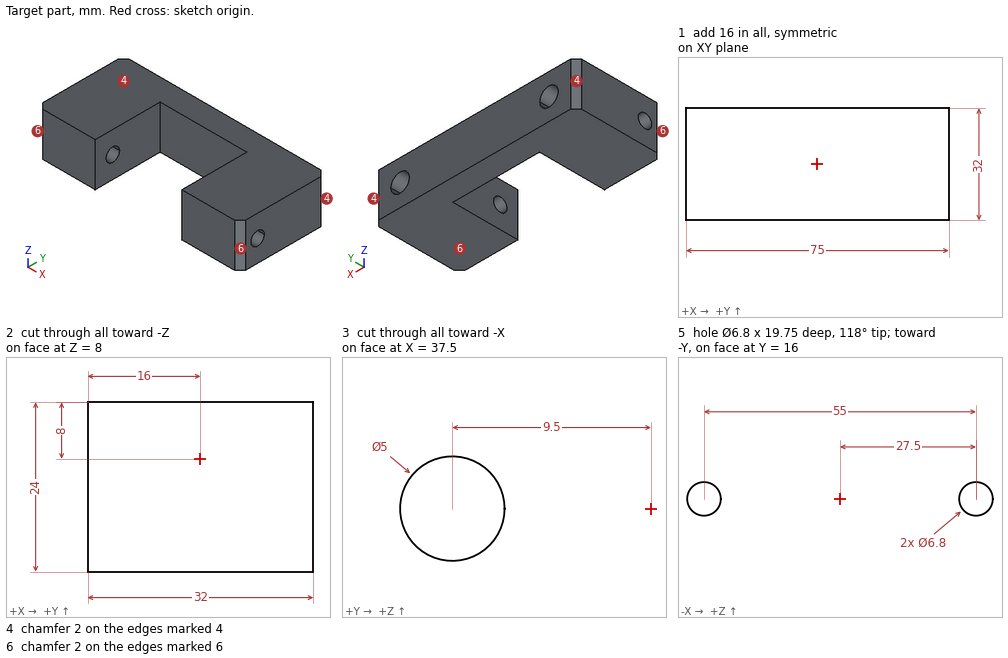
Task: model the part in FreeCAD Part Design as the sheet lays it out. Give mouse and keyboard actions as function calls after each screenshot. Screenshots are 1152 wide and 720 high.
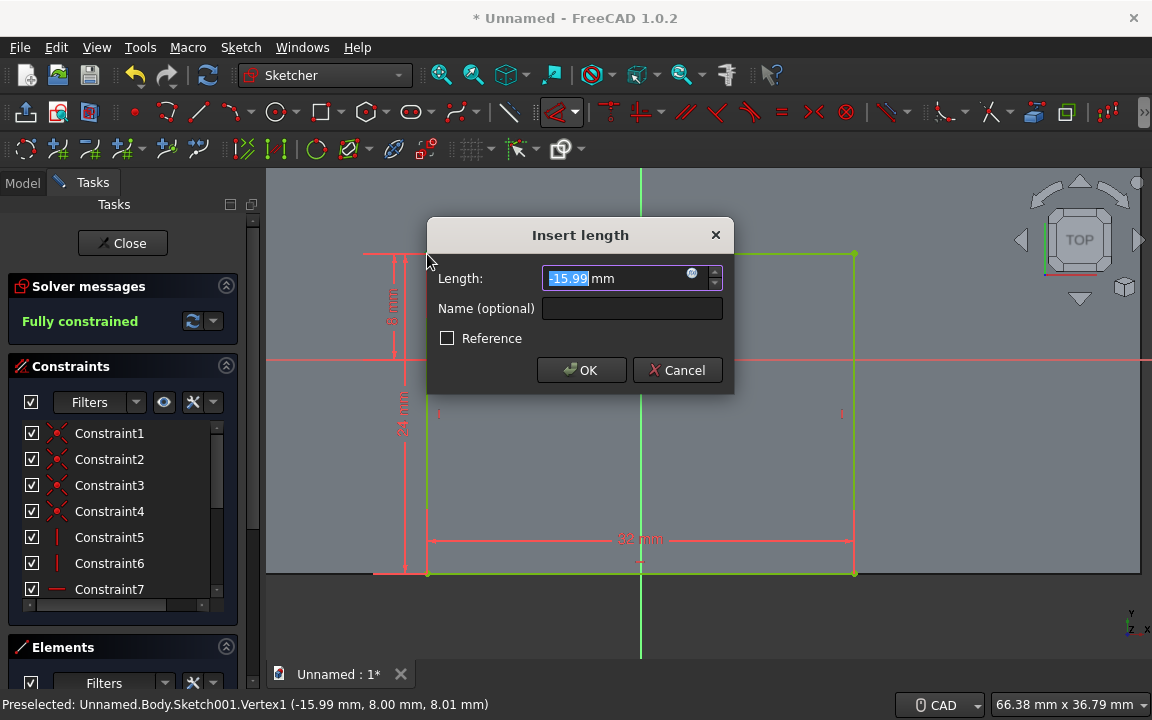
text(-16)
key(Return)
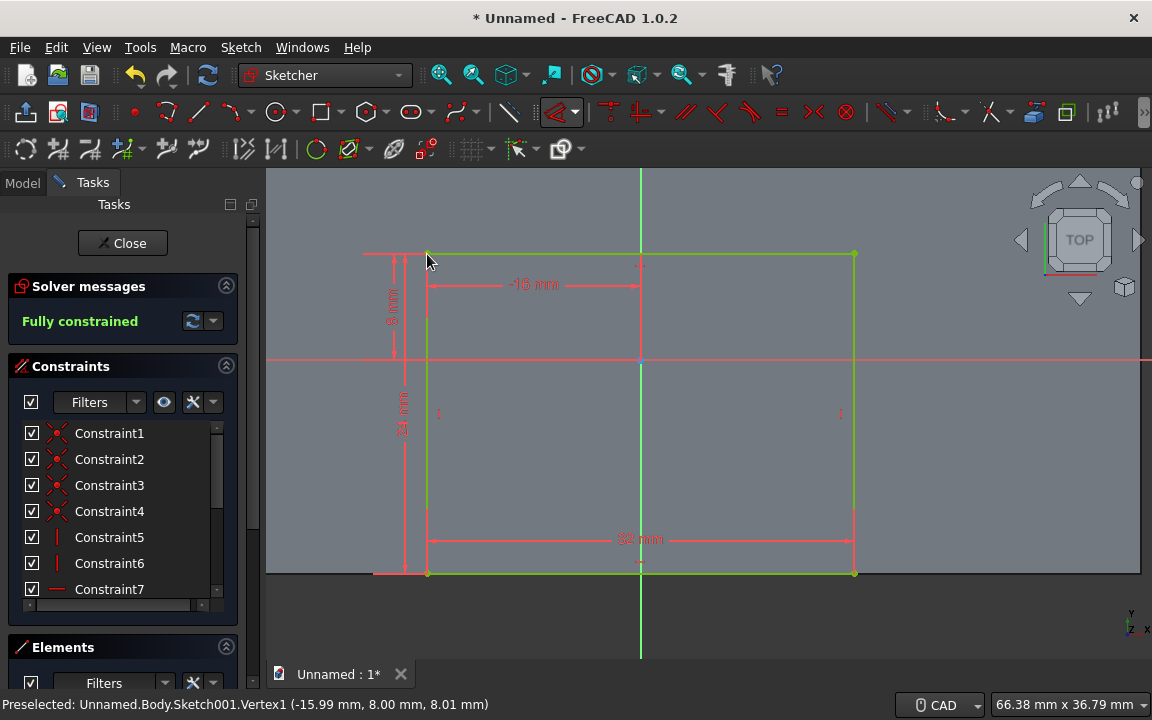
click(123, 243)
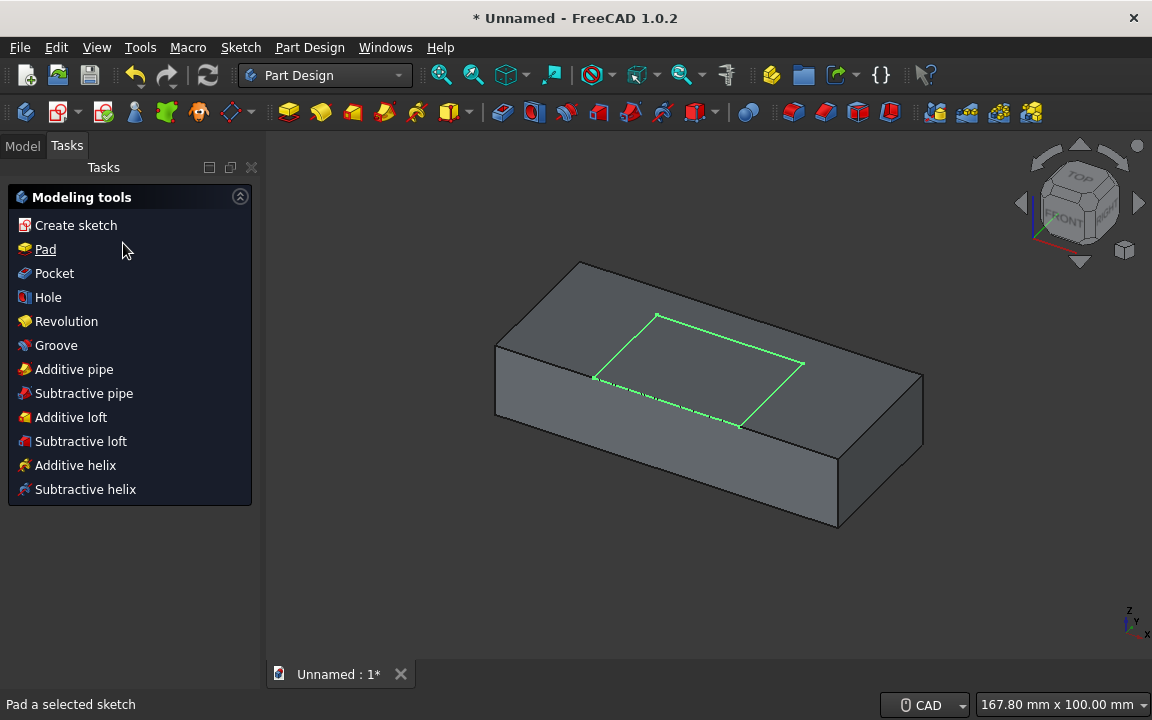
click(504, 112)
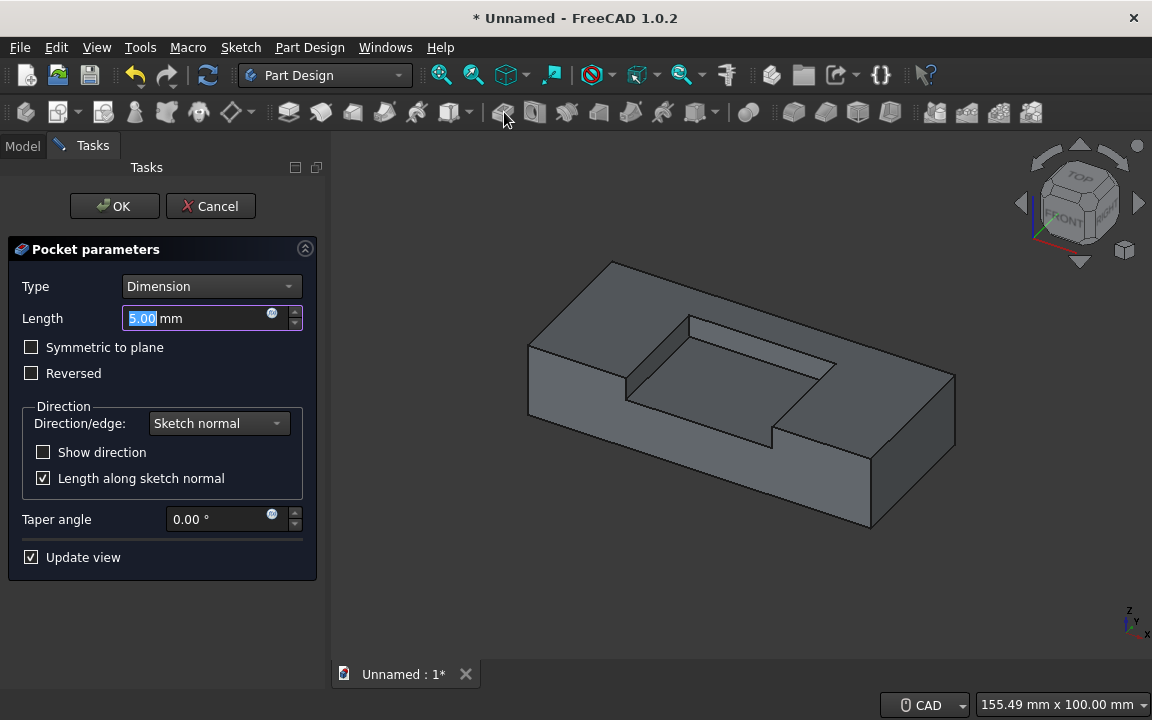
click(212, 286)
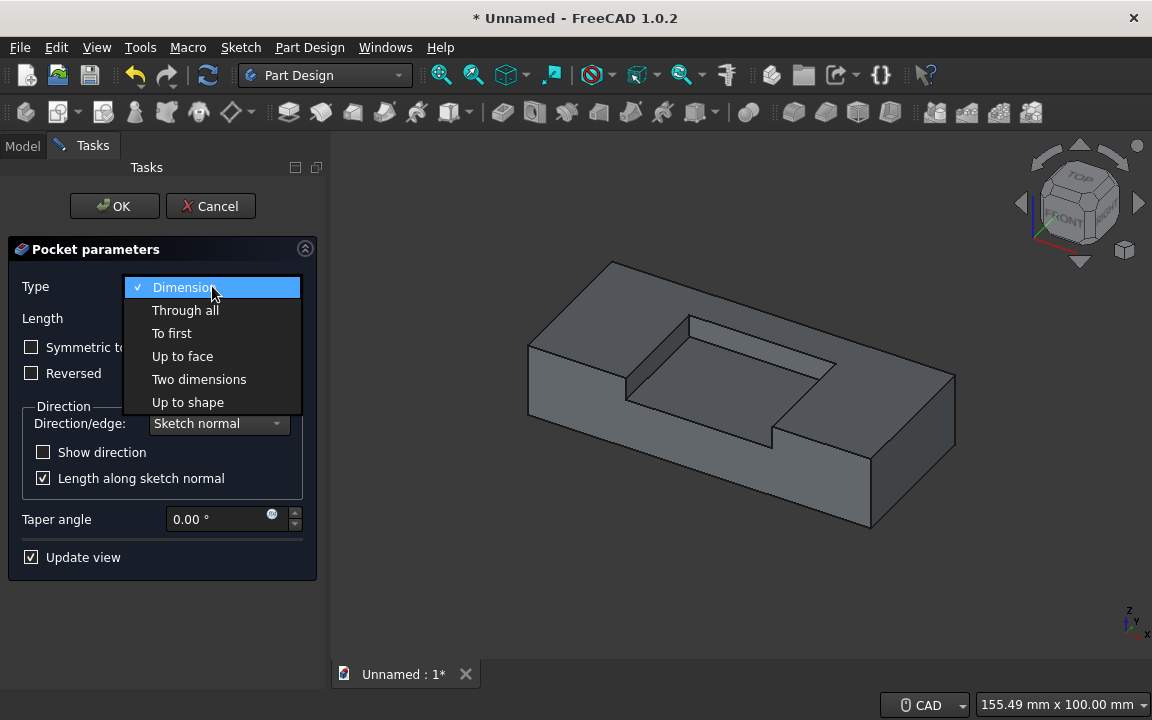
click(212, 310)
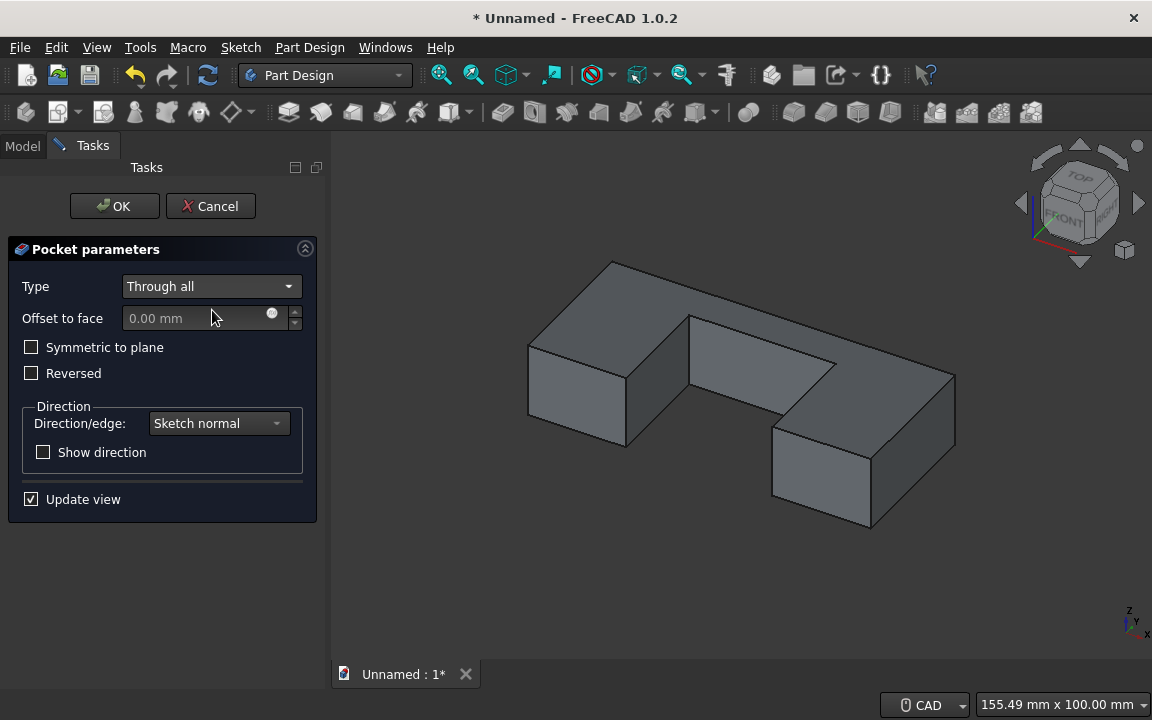
click(115, 206)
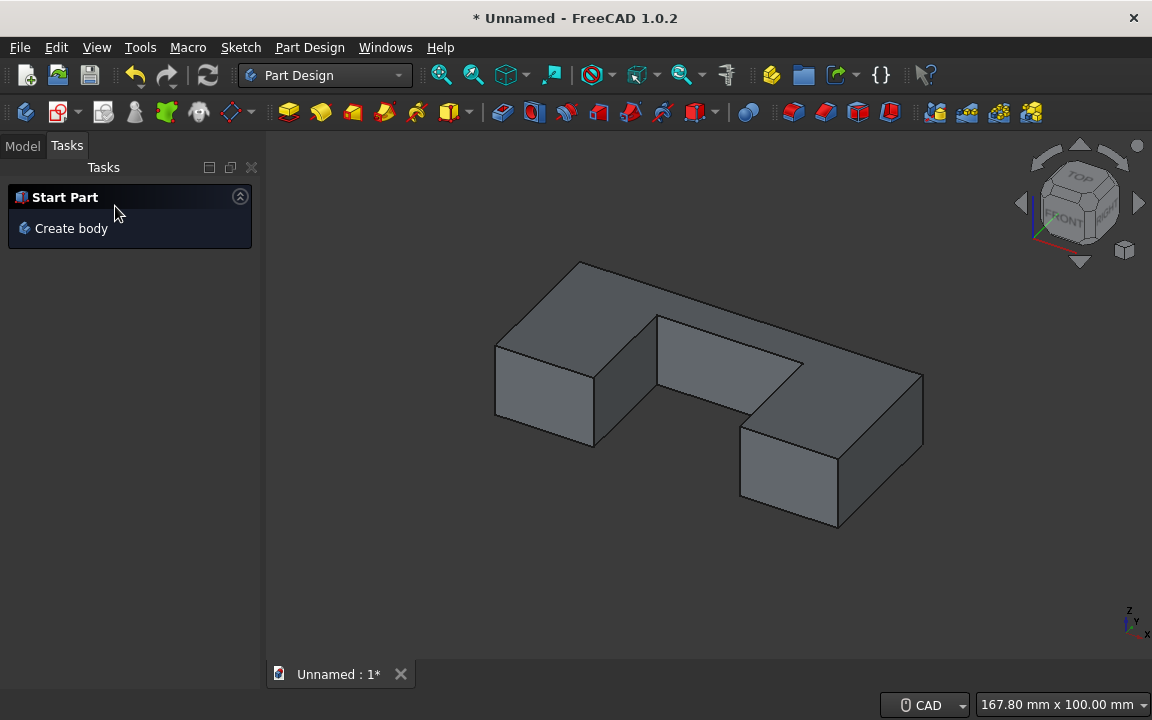
click(893, 439)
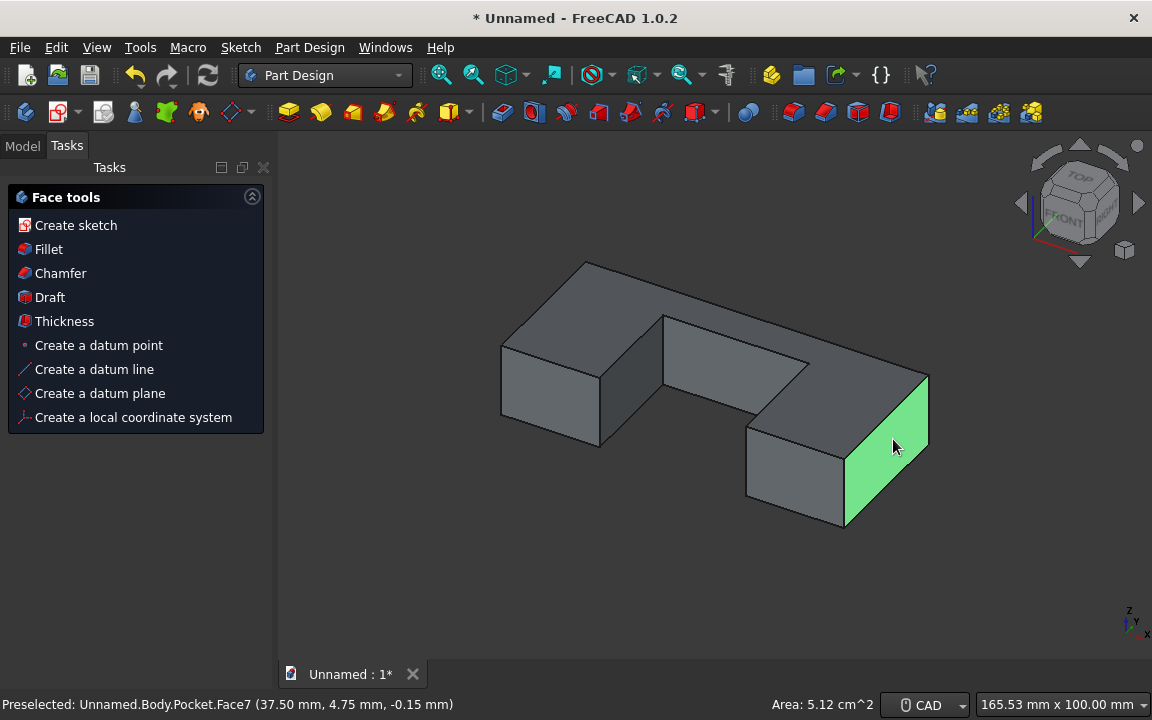
click(58, 112)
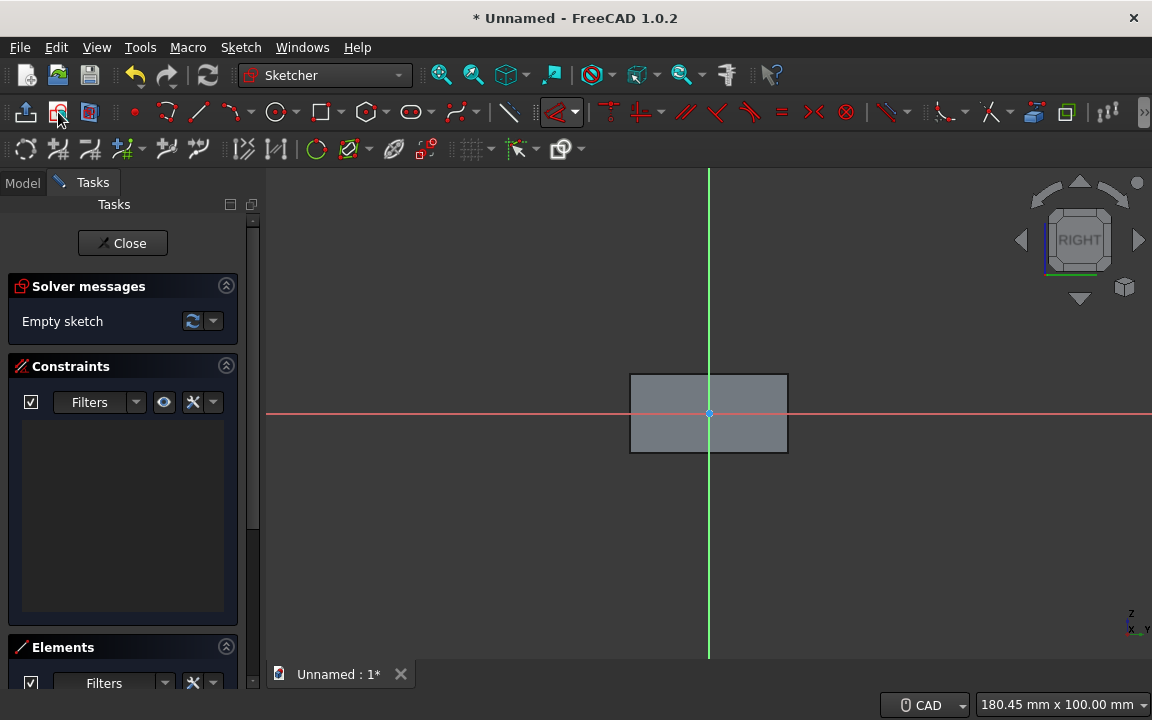
scroll(684, 414, up, 11)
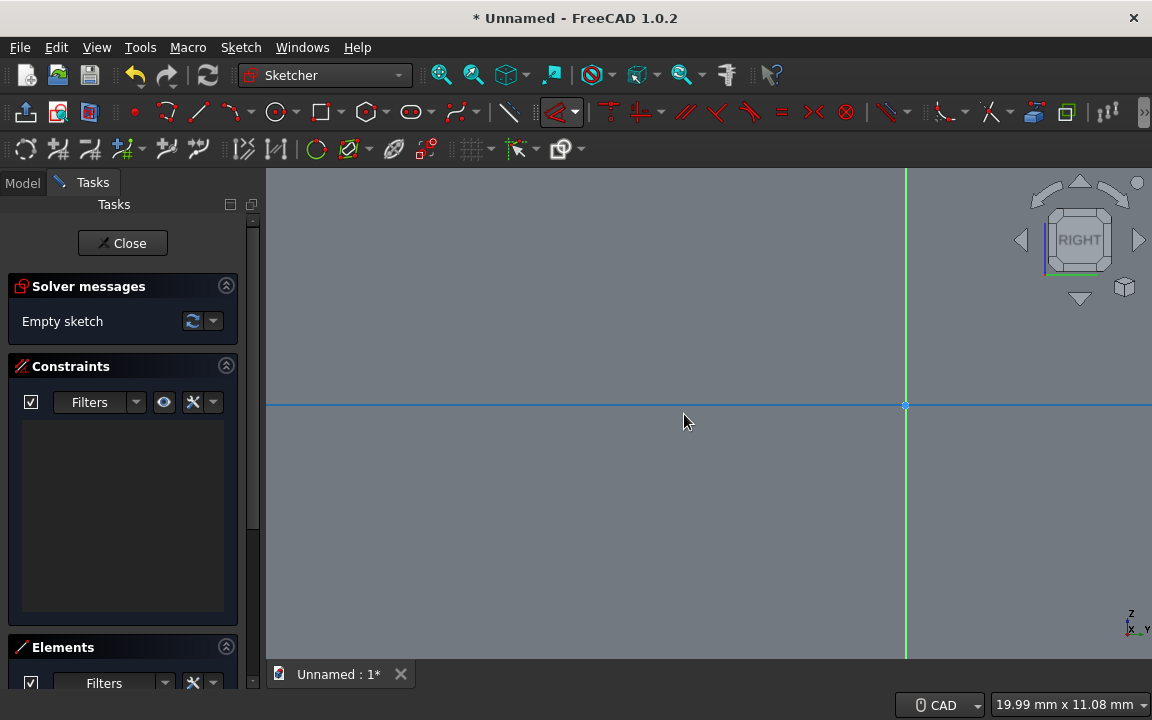
key(g)
key(c)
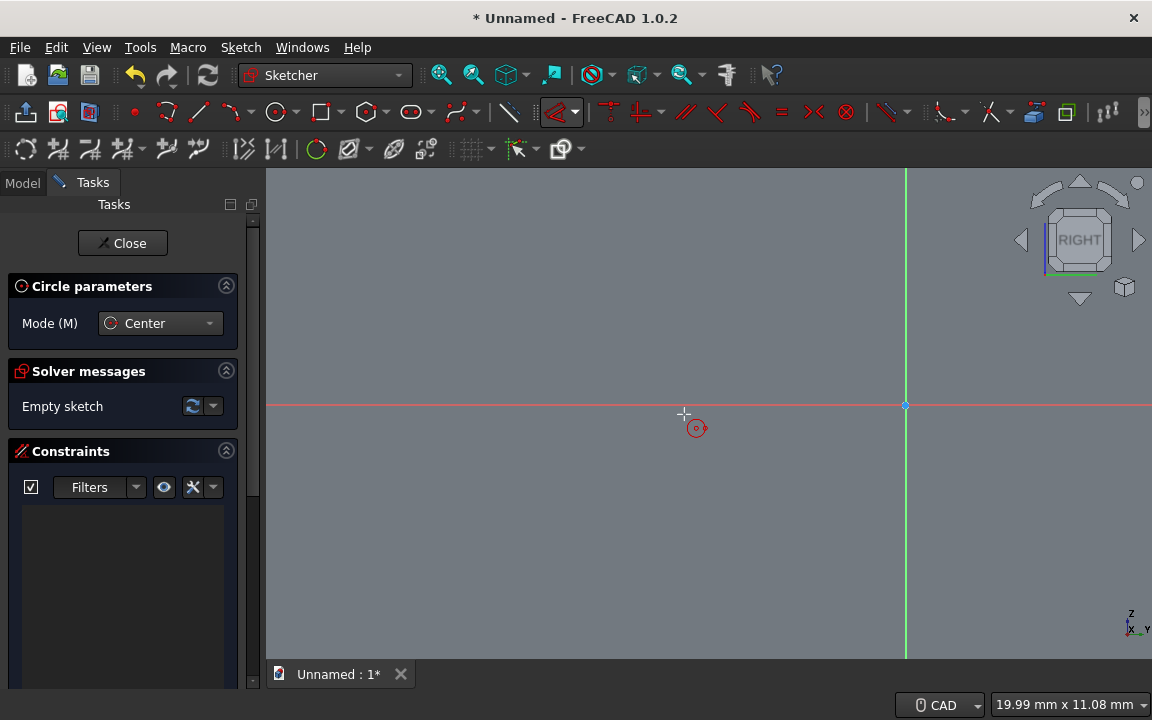
click(485, 405)
click(563, 327)
key(Escape)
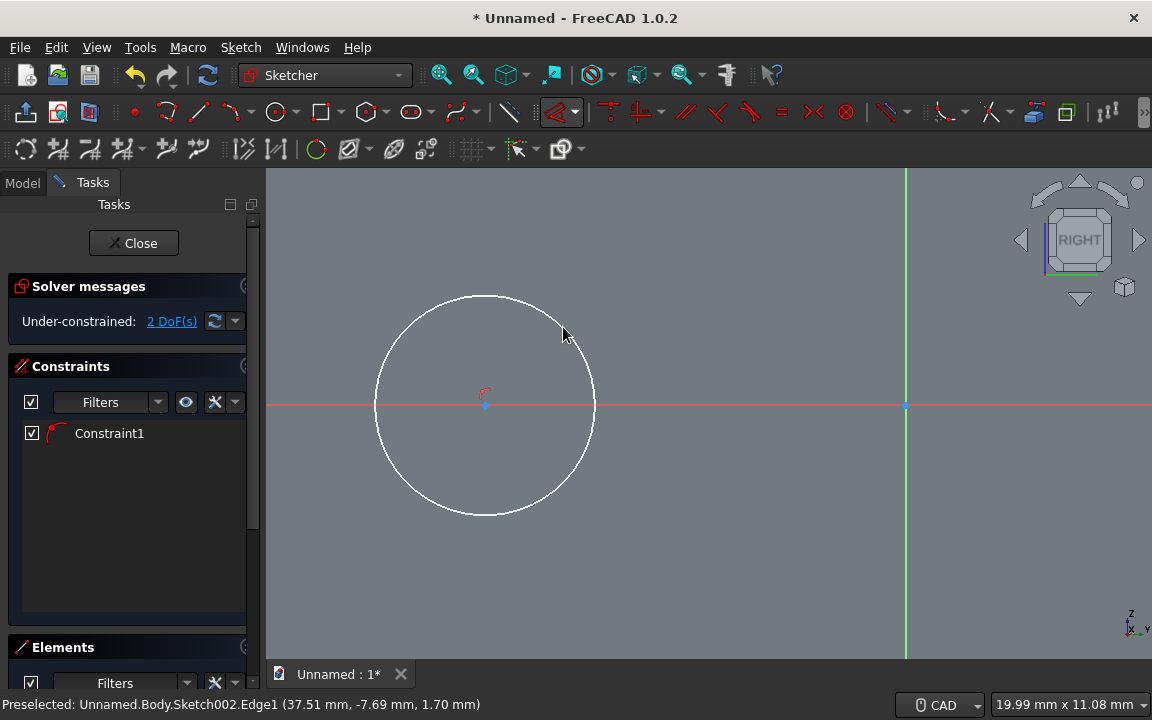
click(562, 327)